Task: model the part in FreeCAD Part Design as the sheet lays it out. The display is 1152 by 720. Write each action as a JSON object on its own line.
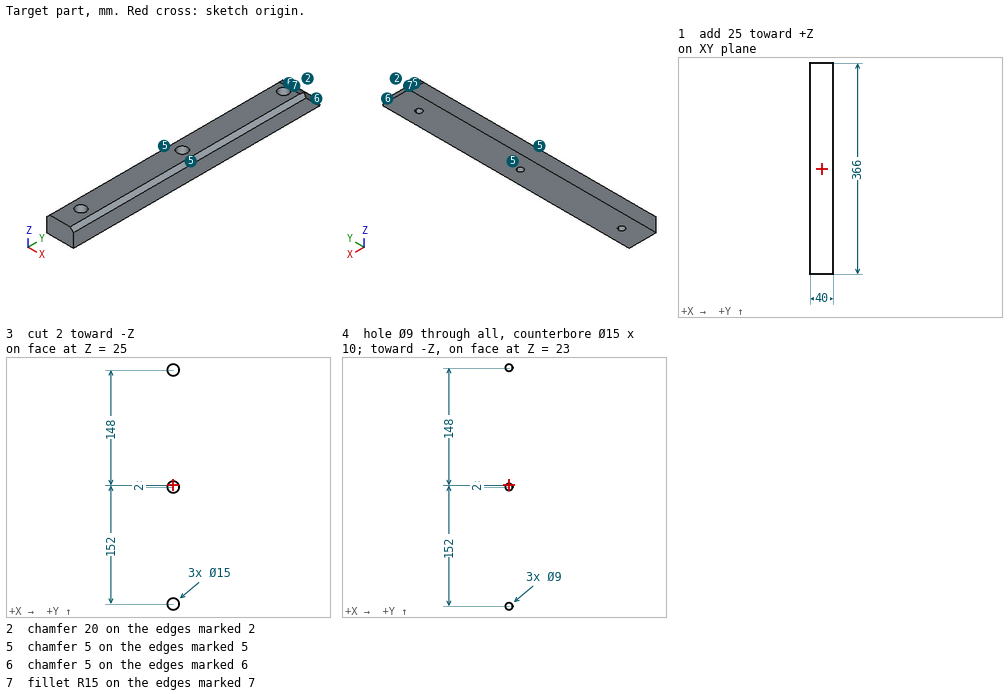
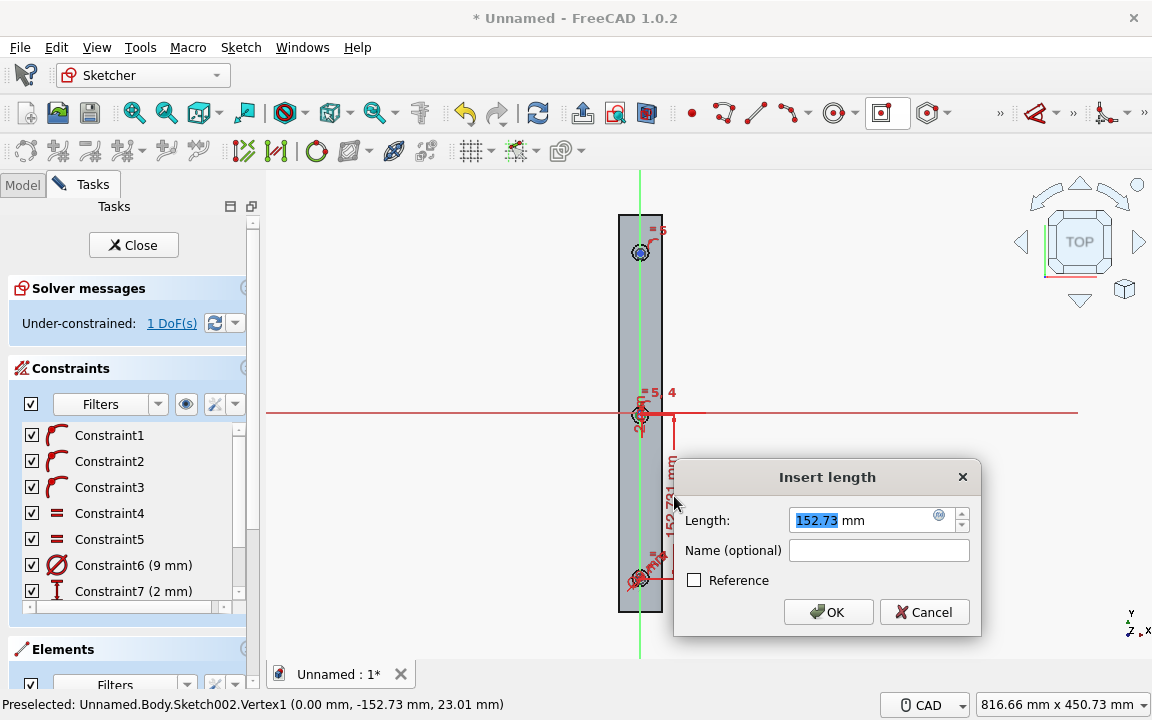
{"action": "type", "text": "152"}
{"action": "key", "text": "Return"}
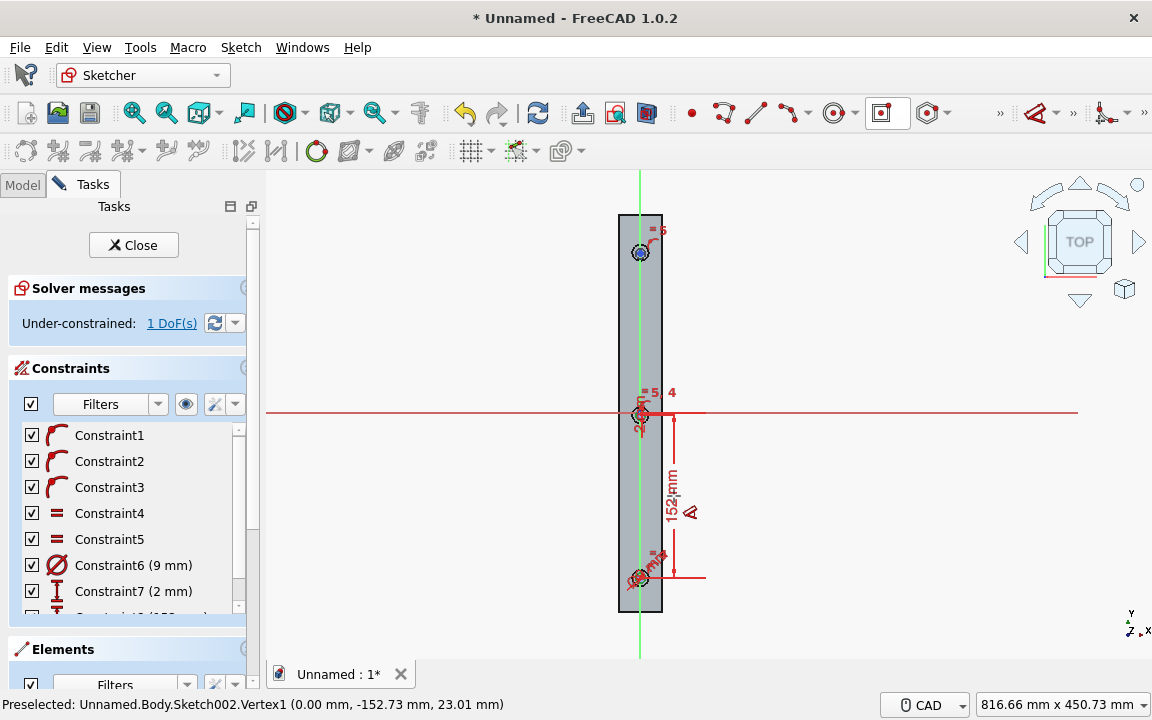
{"action": "left_click", "coordinate": [640, 254]}
{"action": "left_click", "coordinate": [674, 334]}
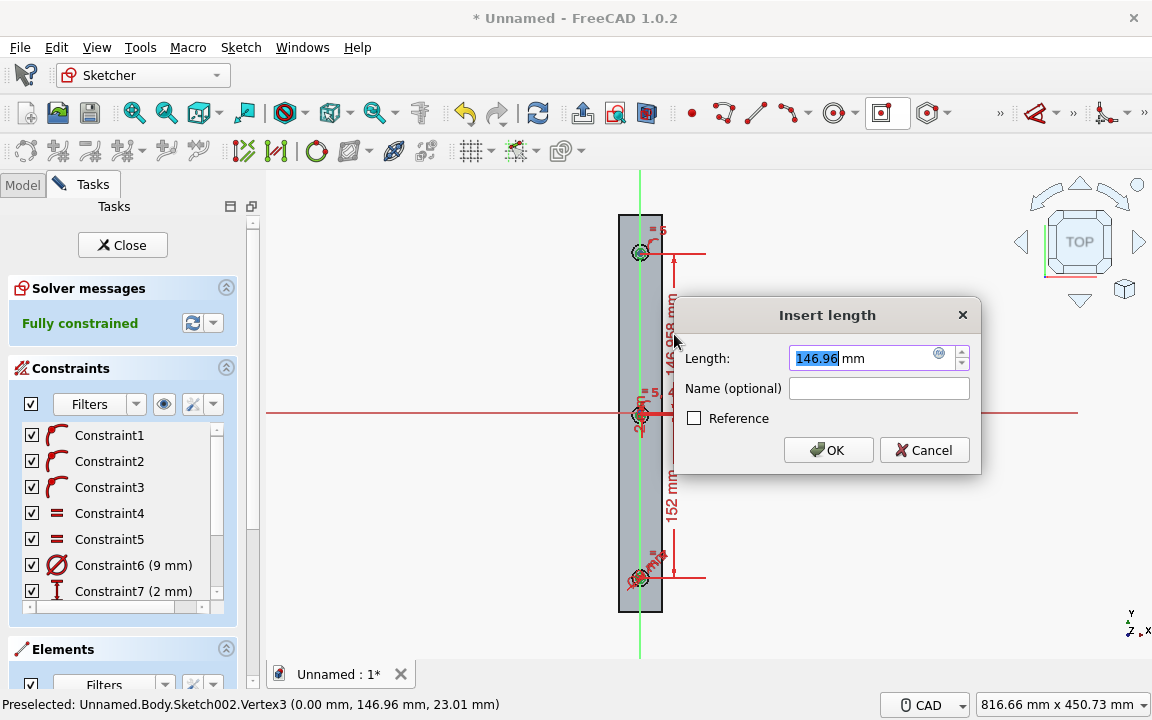
{"action": "type", "text": "148"}
{"action": "key", "text": "Return"}
{"action": "key", "text": "Escape"}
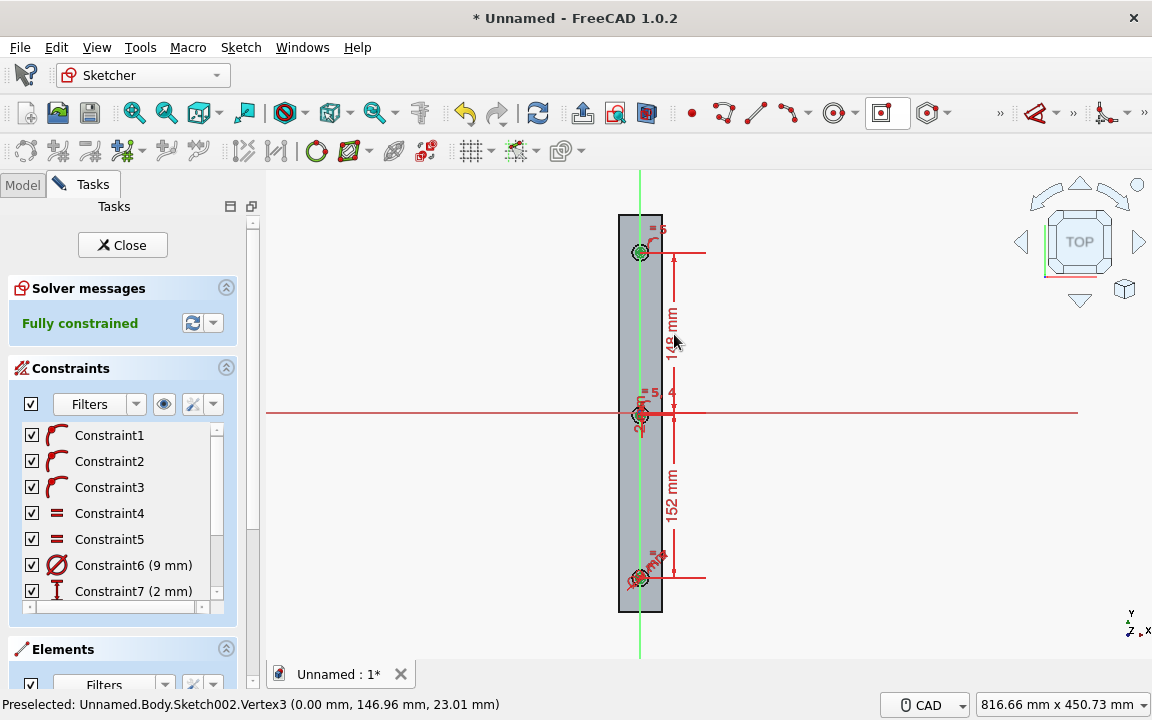
{"action": "left_click", "coordinate": [123, 245]}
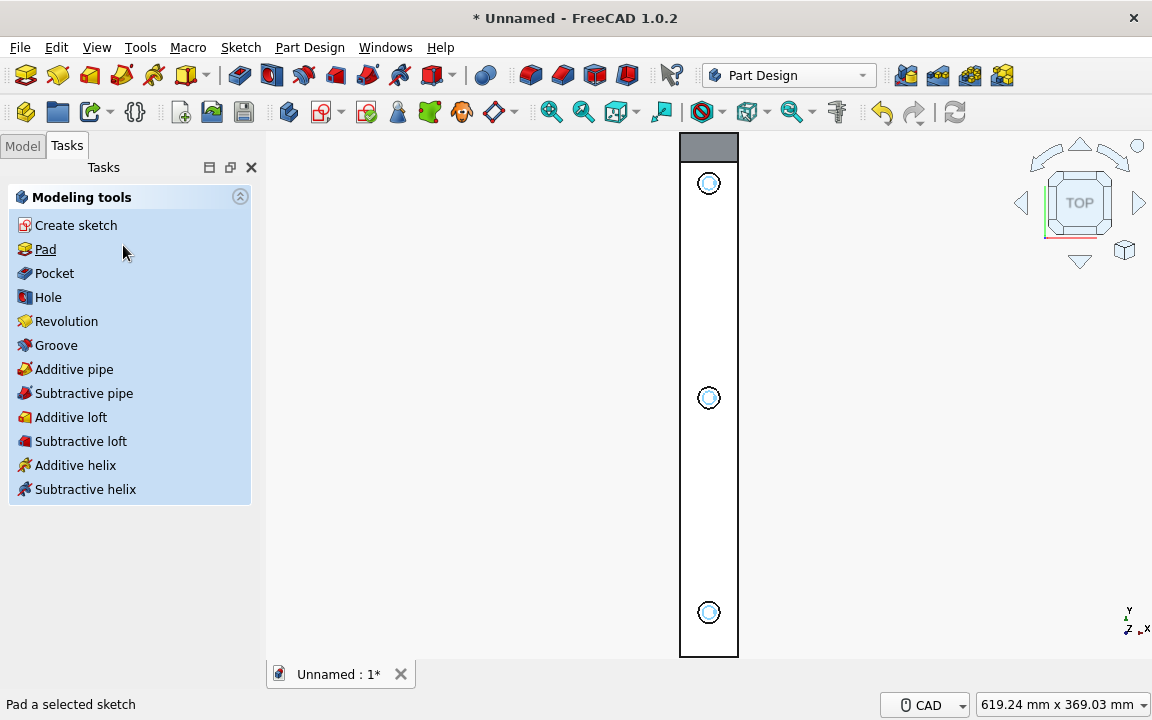
{"action": "left_click", "coordinate": [272, 76]}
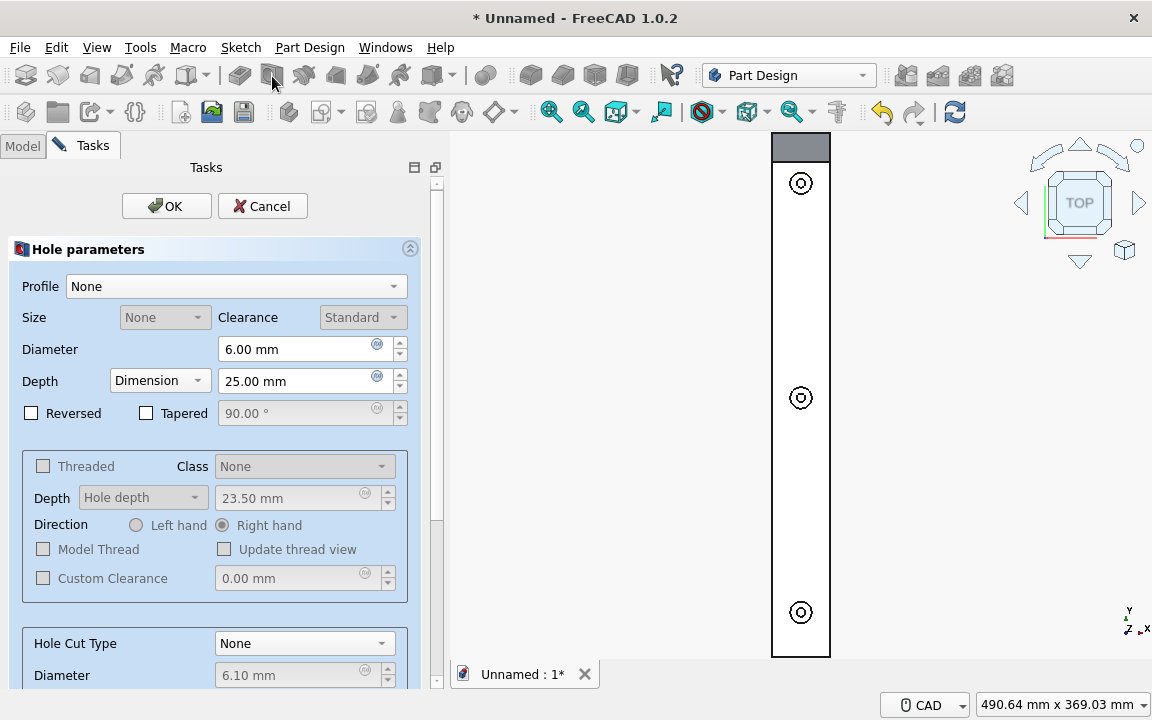
{"action": "triple_click", "coordinate": [305, 349]}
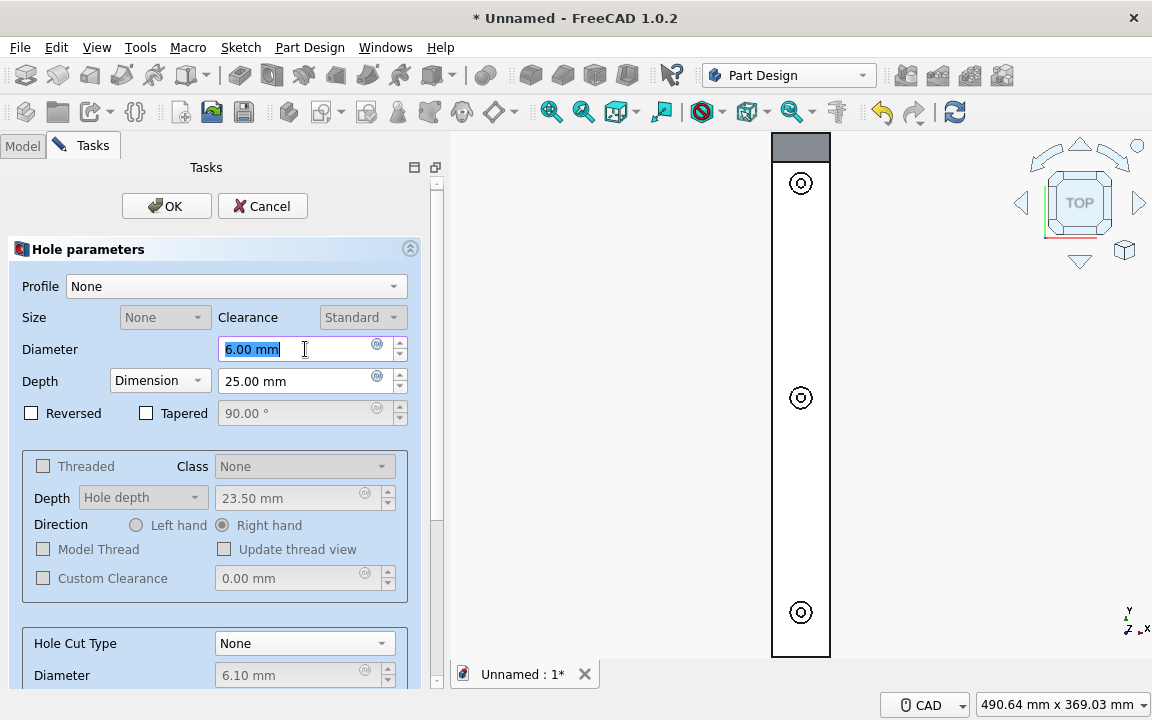
{"action": "type", "text": "9"}
{"action": "key", "text": "Tab"}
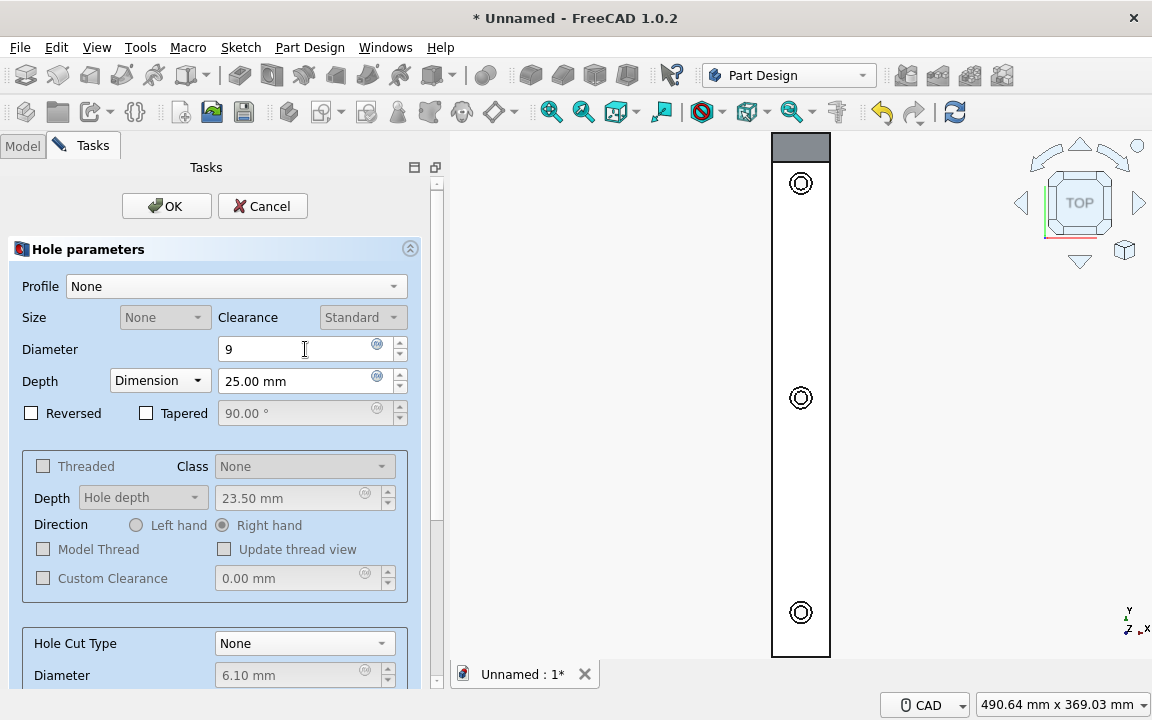
{"action": "left_click", "coordinate": [161, 380]}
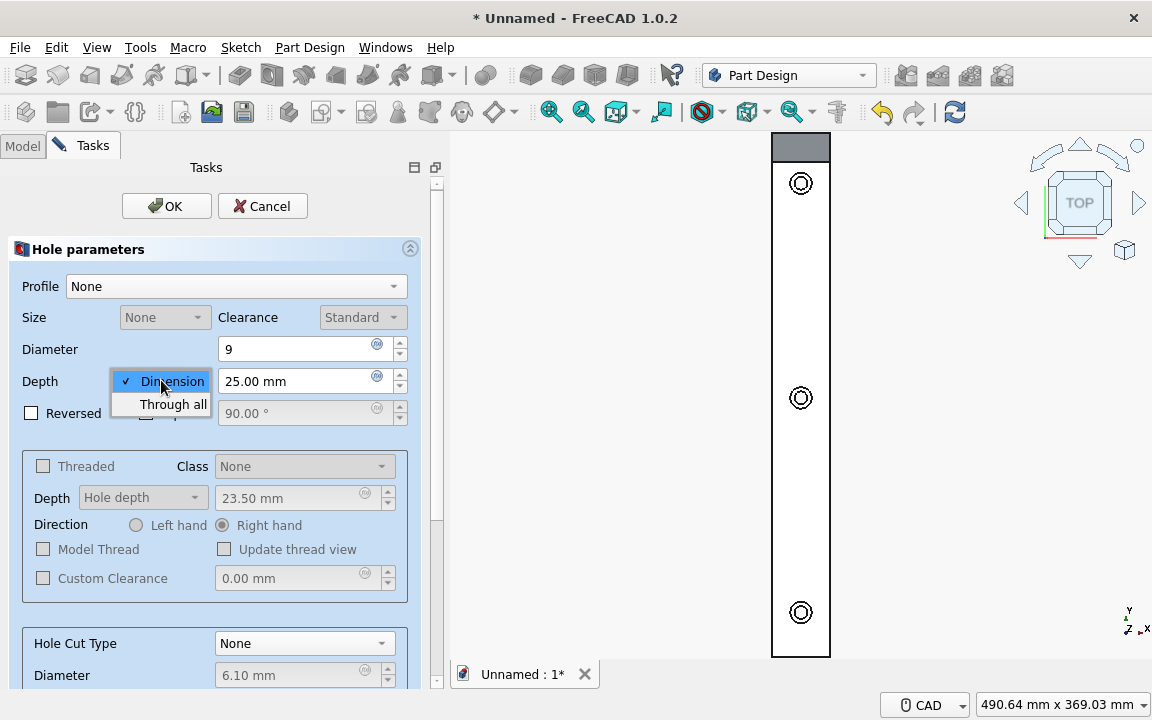
{"action": "left_click", "coordinate": [160, 404]}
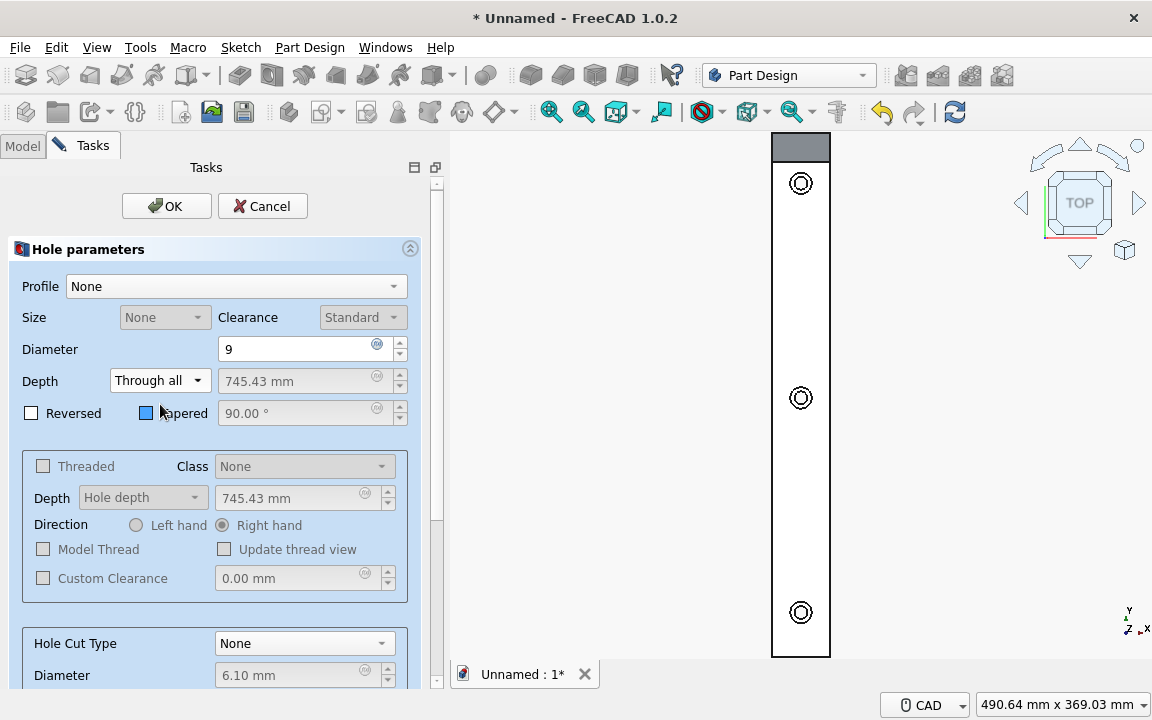
{"action": "left_click", "coordinate": [306, 644]}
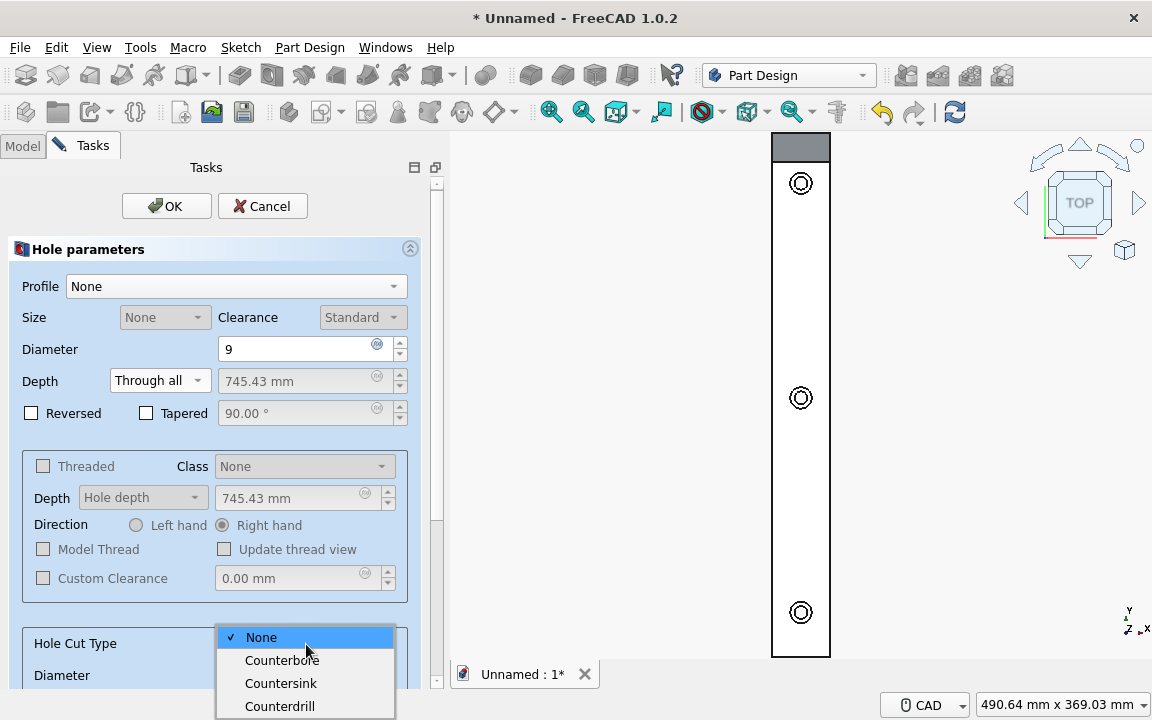
{"action": "left_click", "coordinate": [304, 660]}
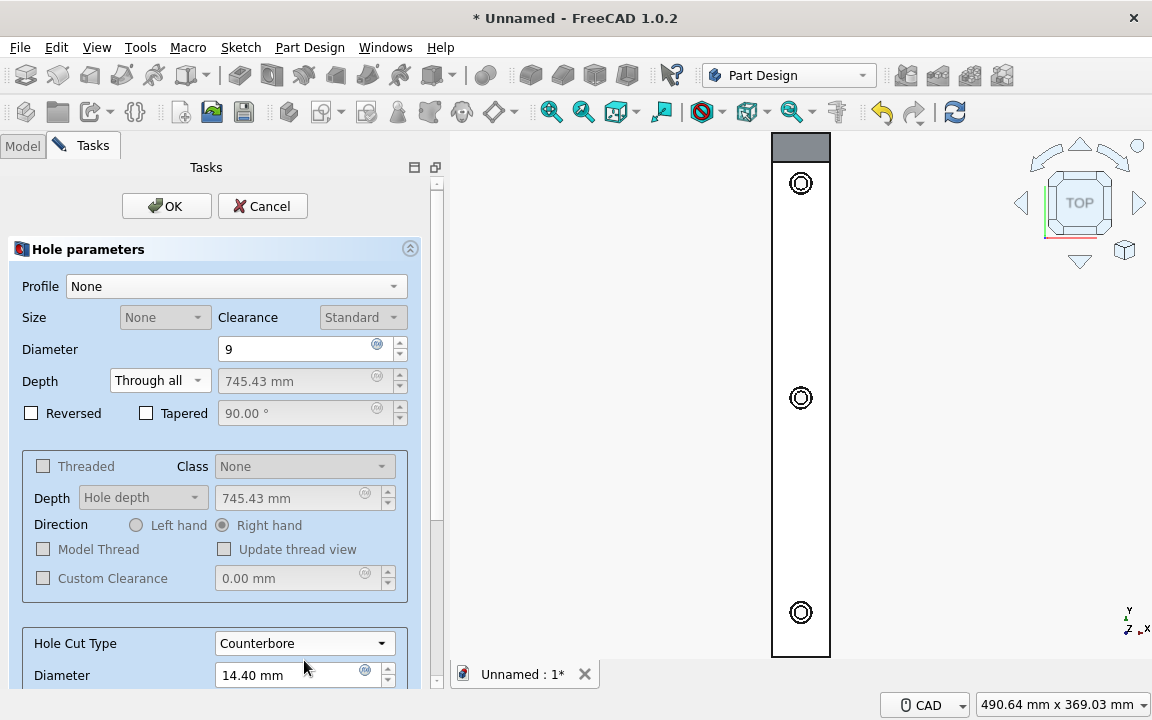
{"action": "triple_click", "coordinate": [298, 675]}